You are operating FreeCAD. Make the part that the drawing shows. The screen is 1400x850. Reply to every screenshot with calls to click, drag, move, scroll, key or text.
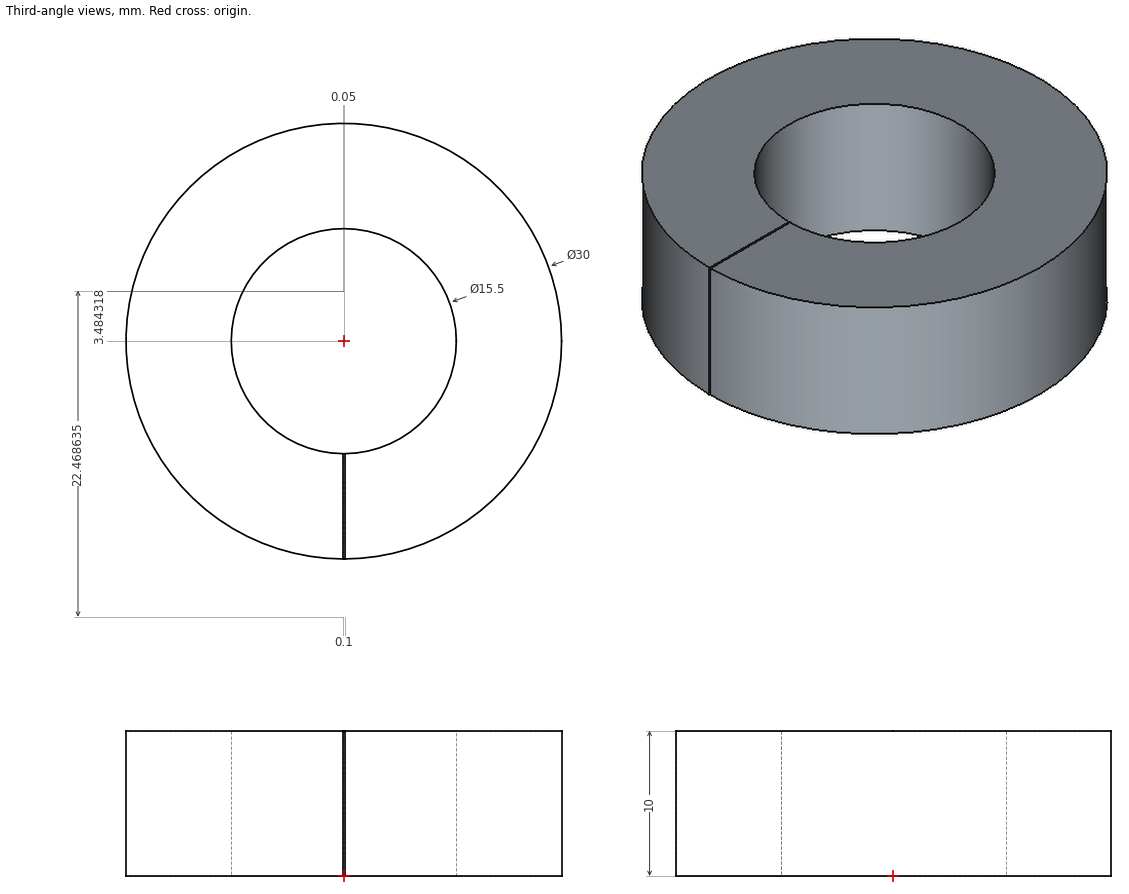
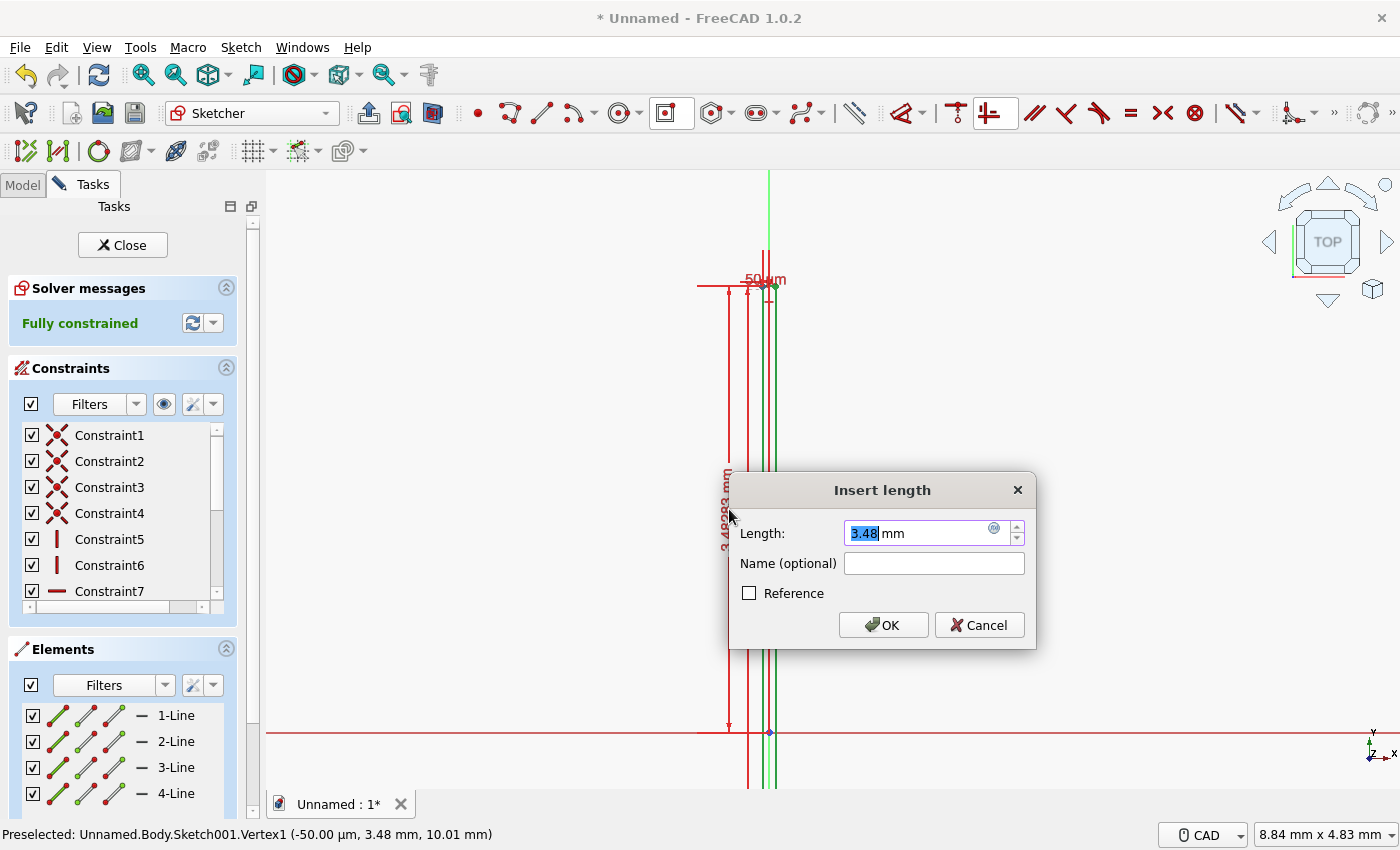
text(3.484318)
key(Return)
key(Escape)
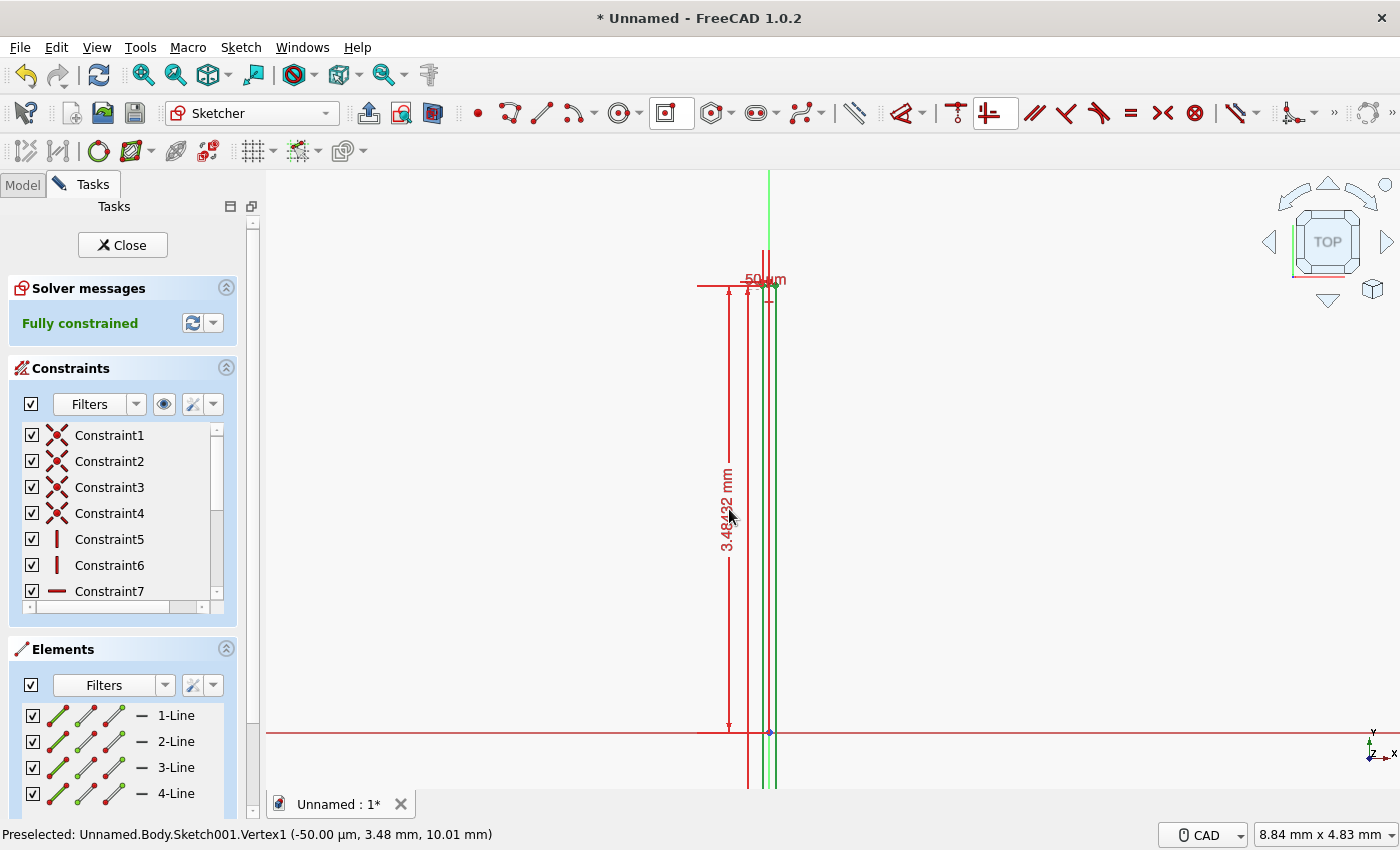
click(123, 245)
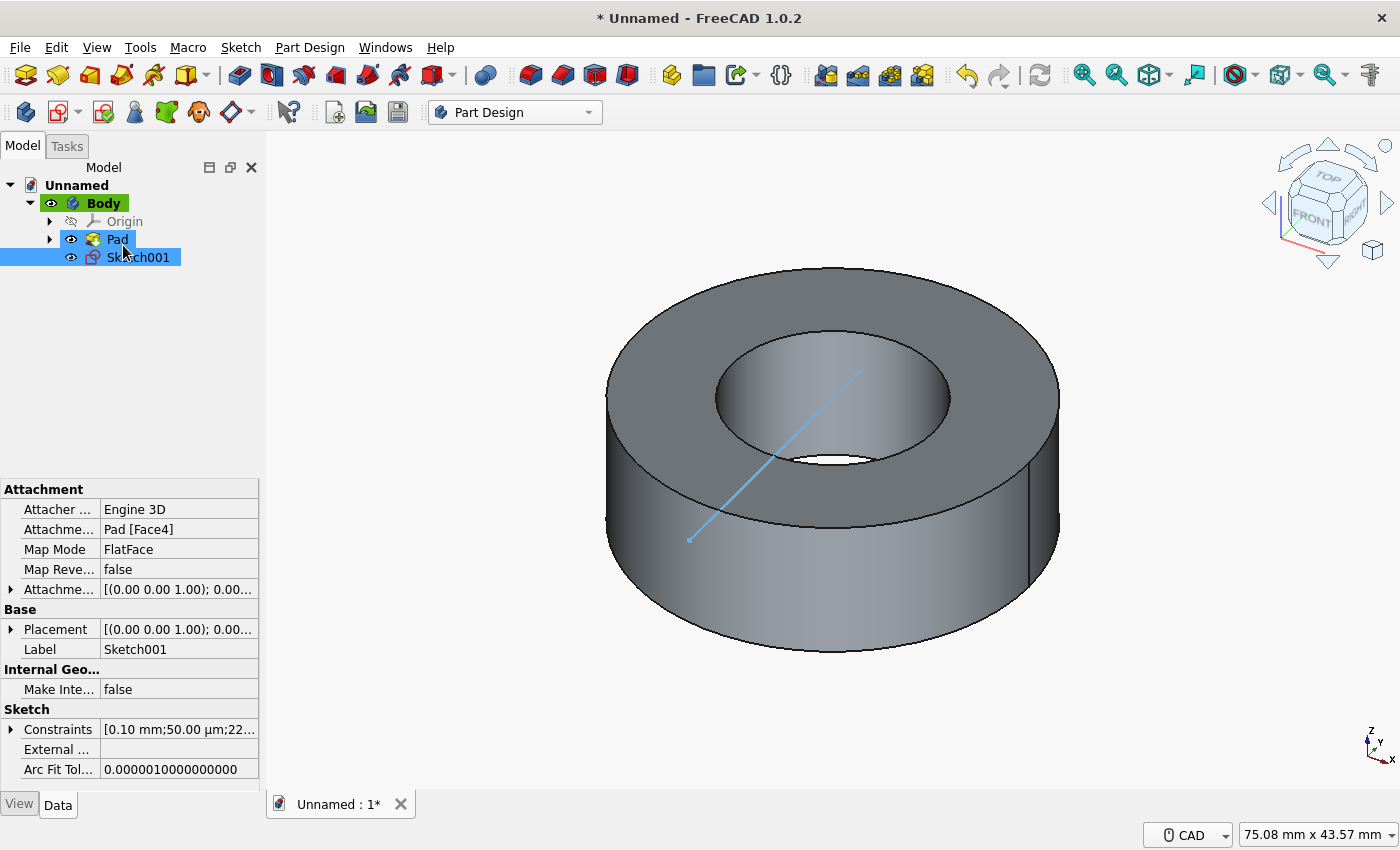
click(240, 76)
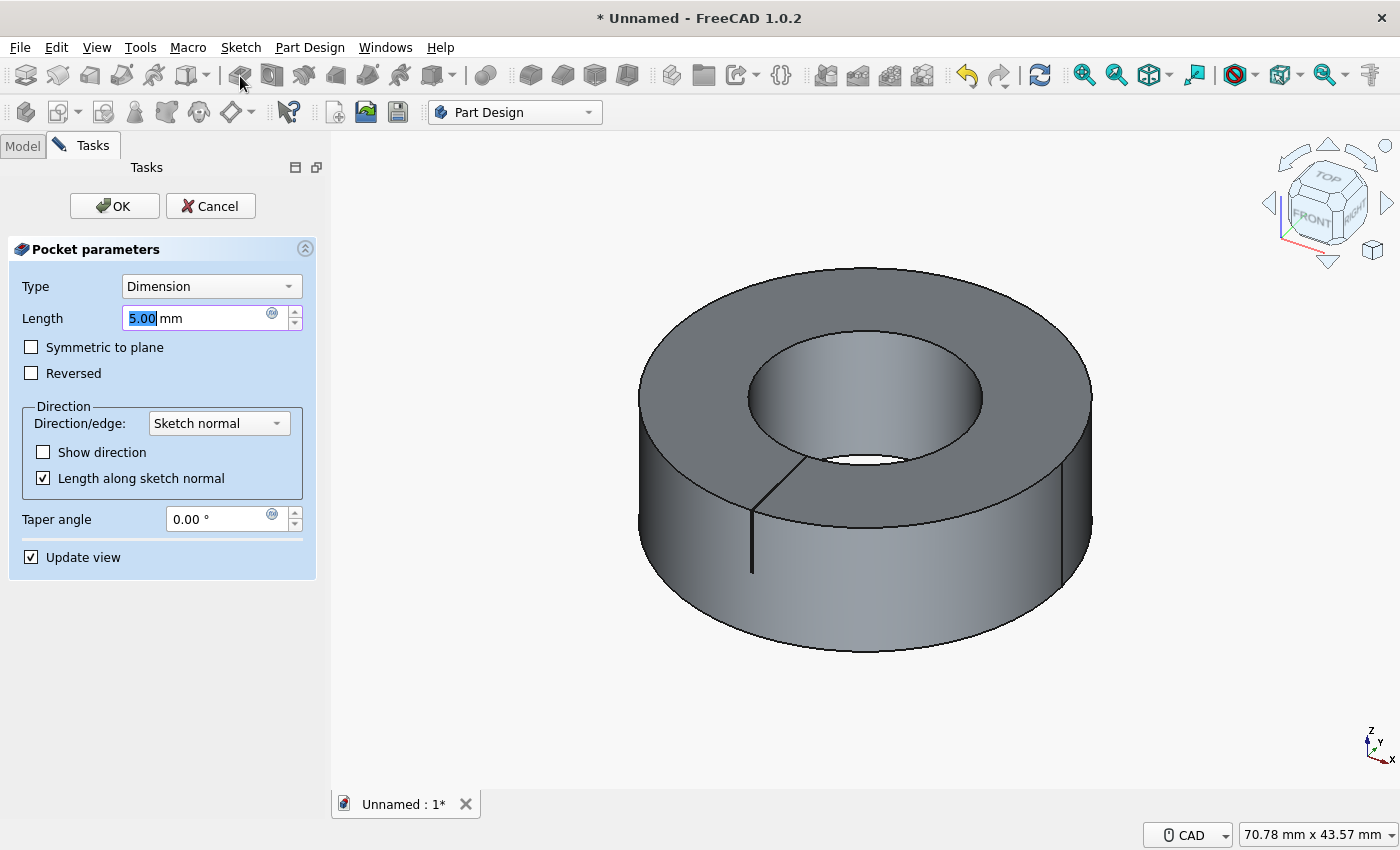
click(212, 286)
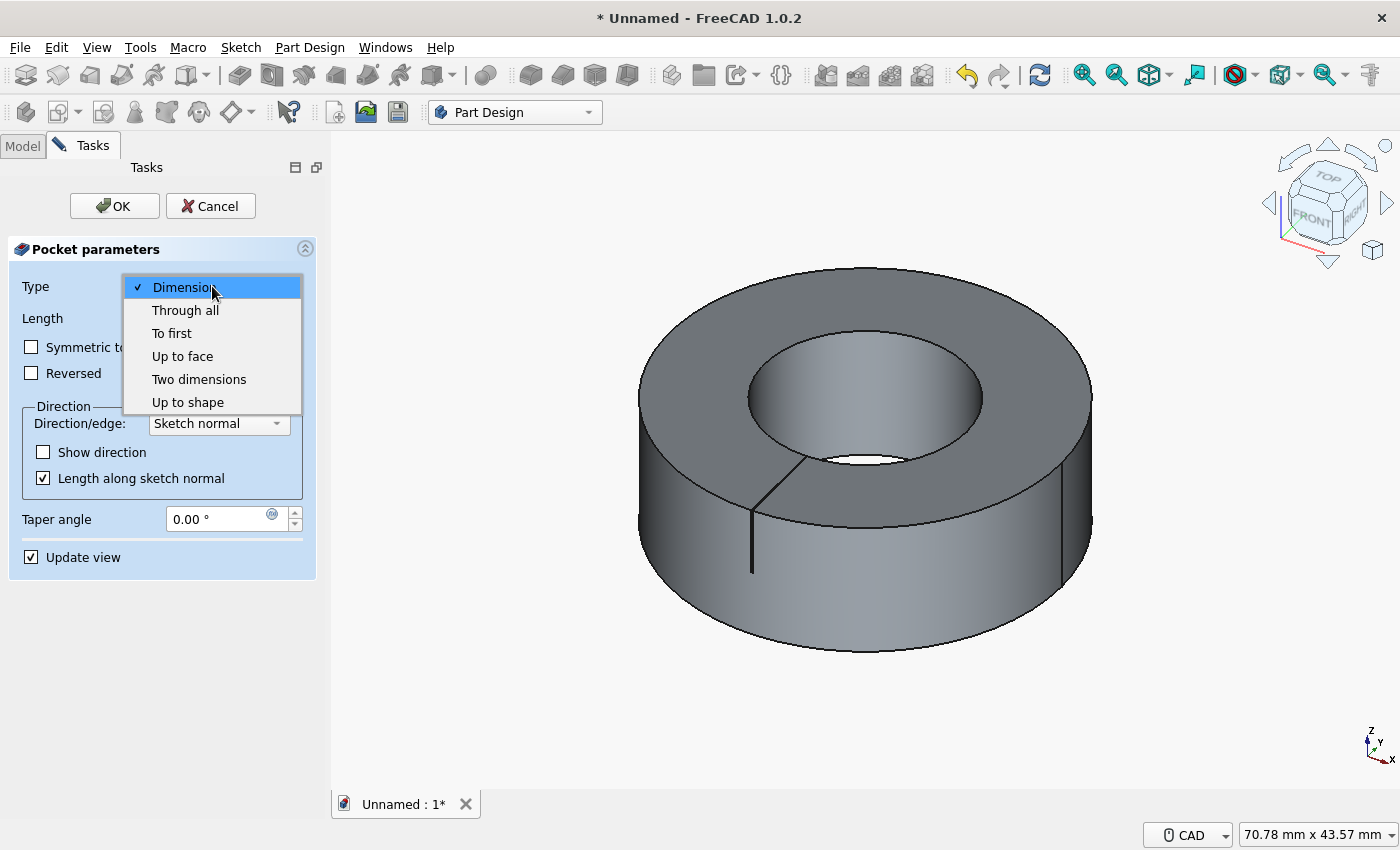
click(212, 310)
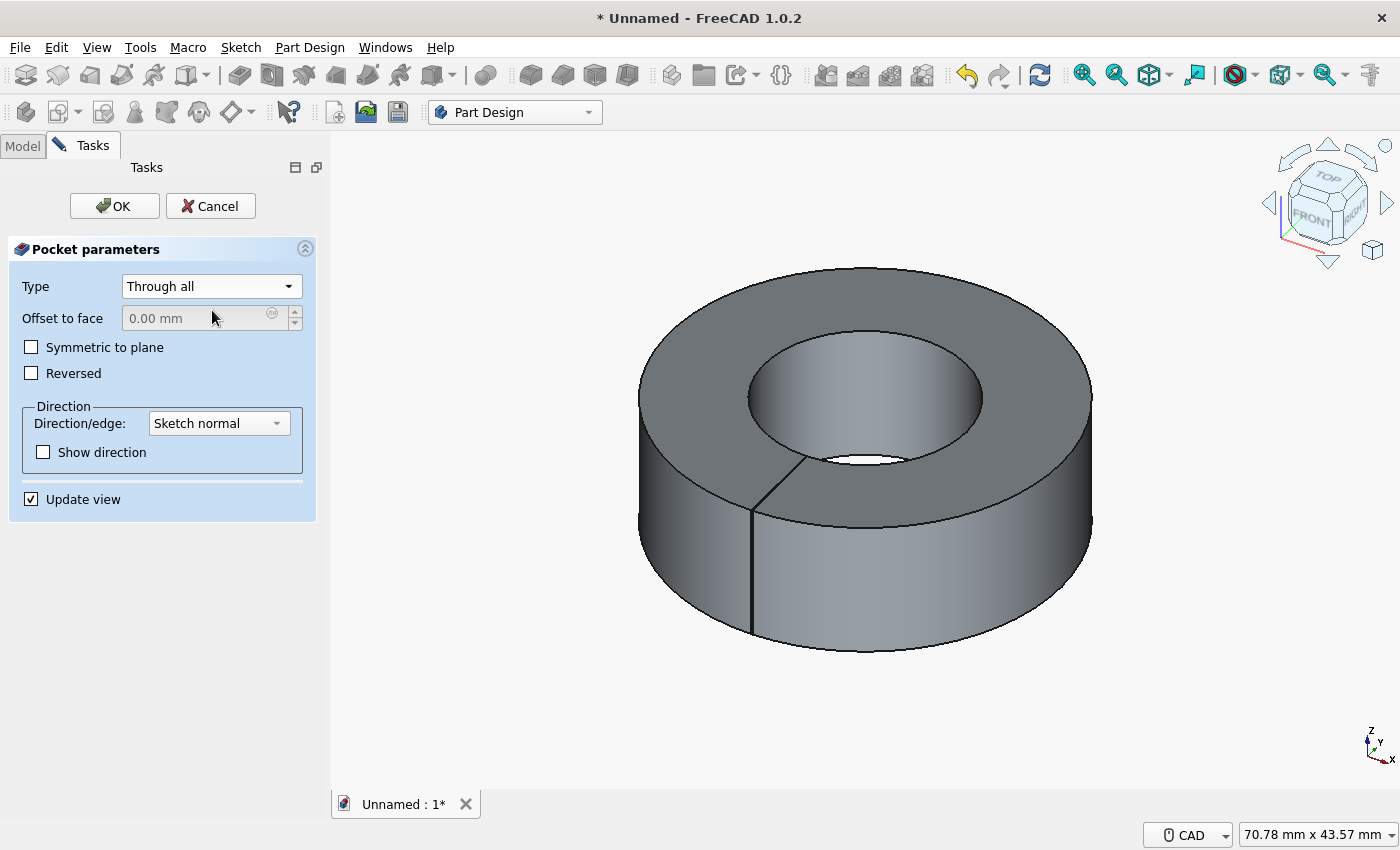
click(115, 206)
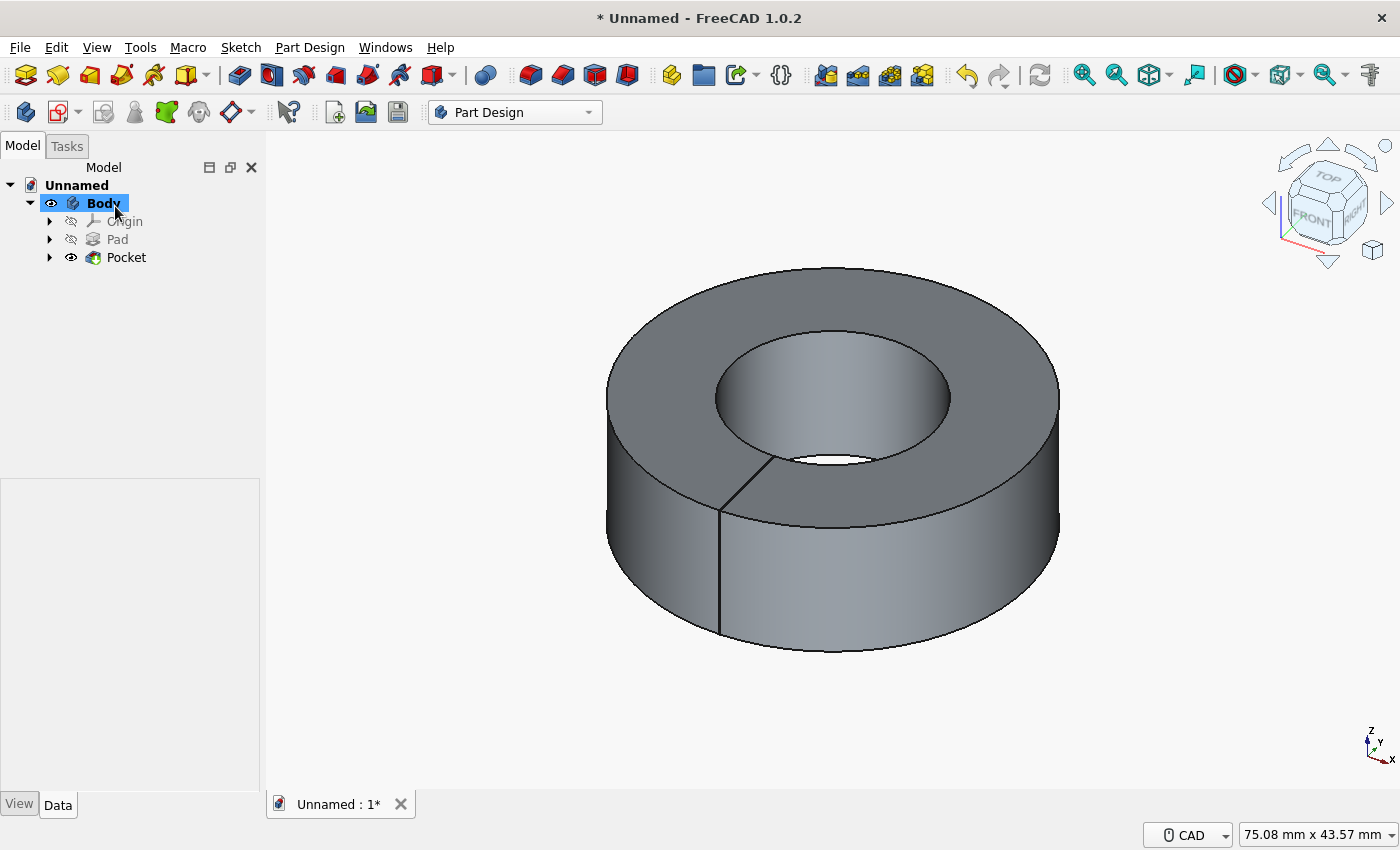
key(0)